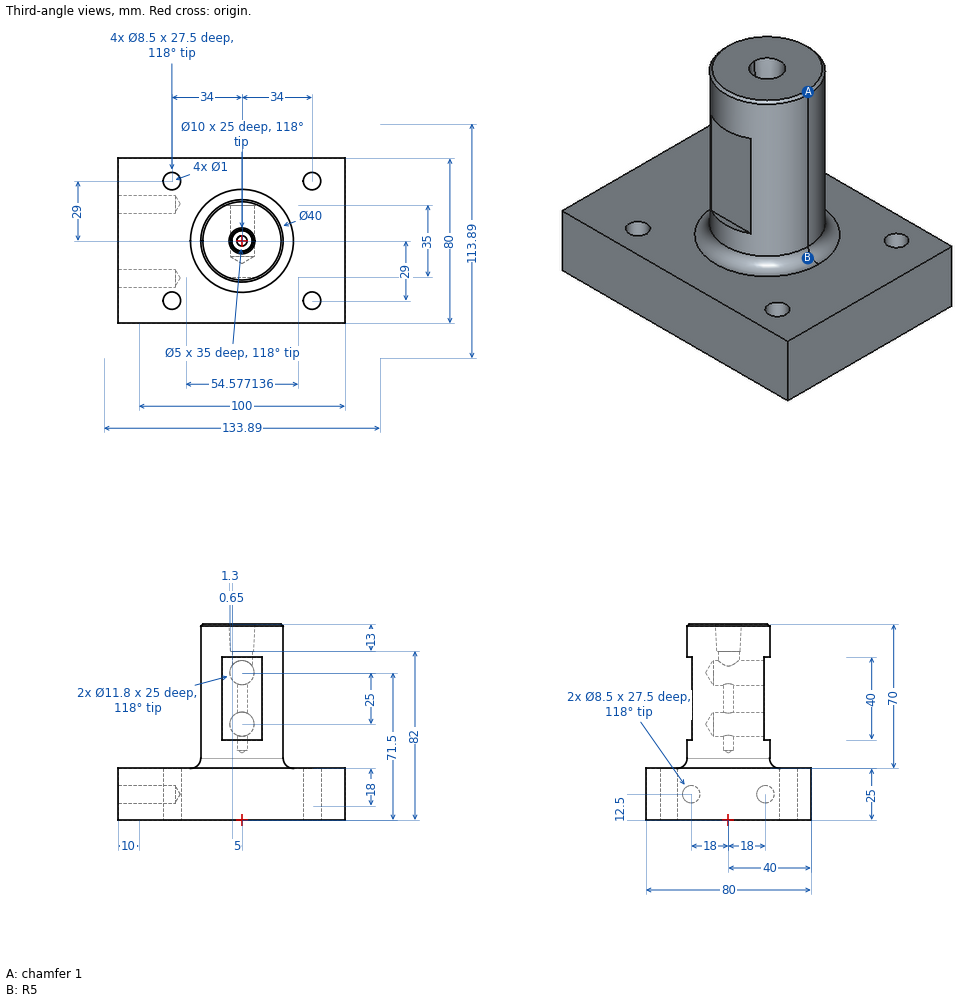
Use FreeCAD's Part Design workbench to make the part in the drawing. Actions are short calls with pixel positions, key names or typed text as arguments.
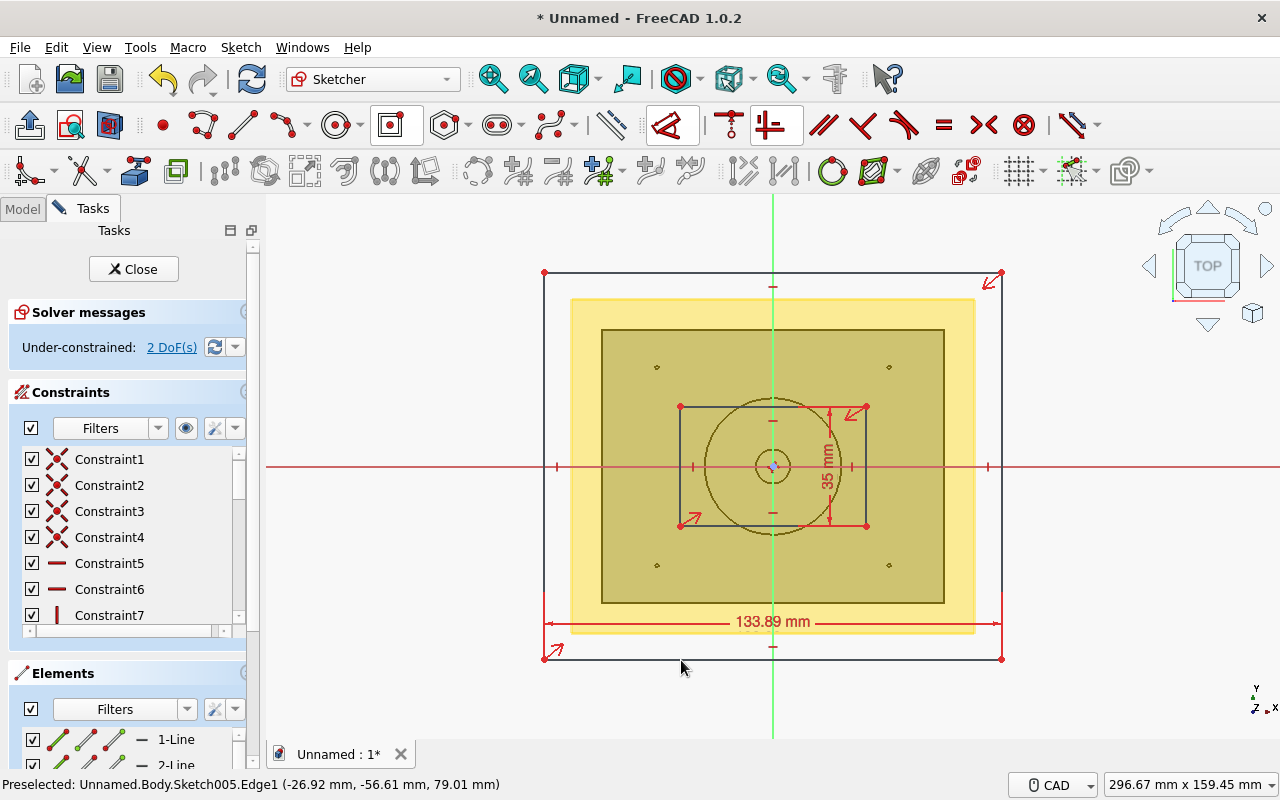
click(1002, 544)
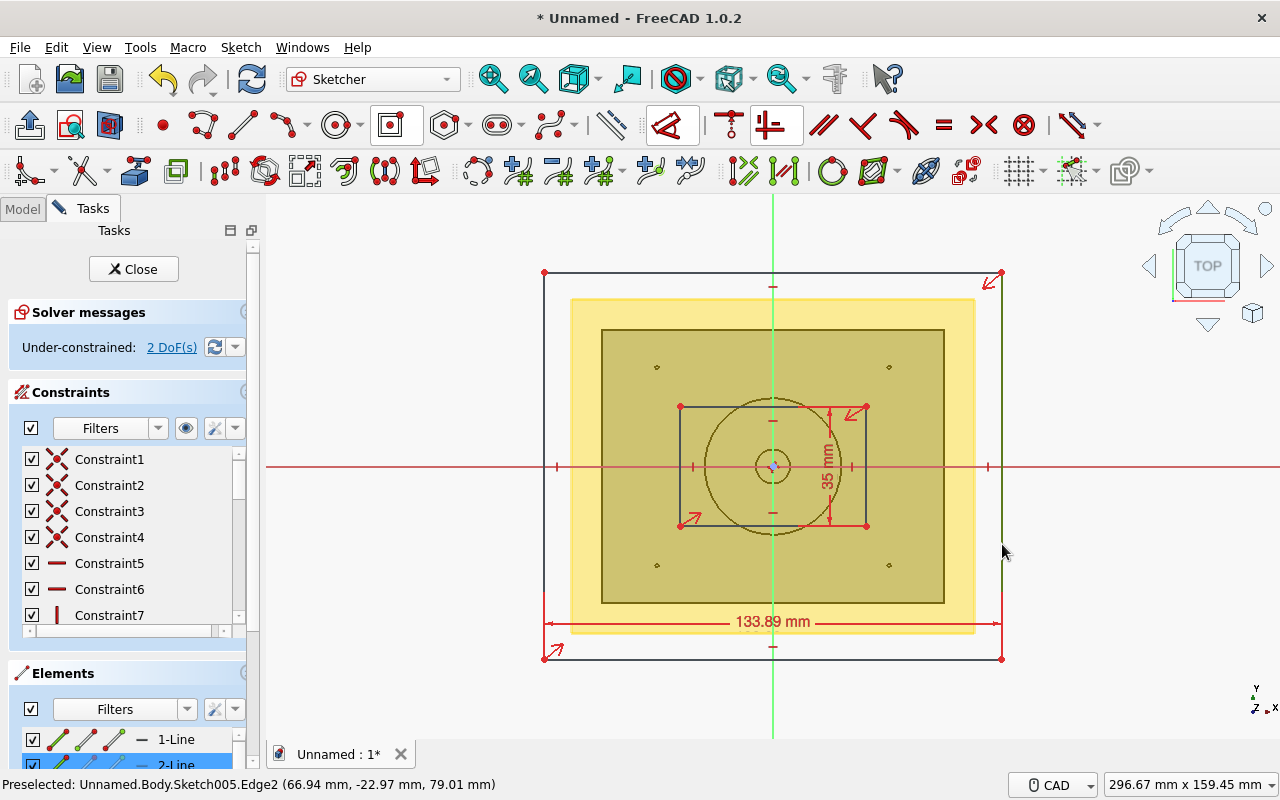
key(i)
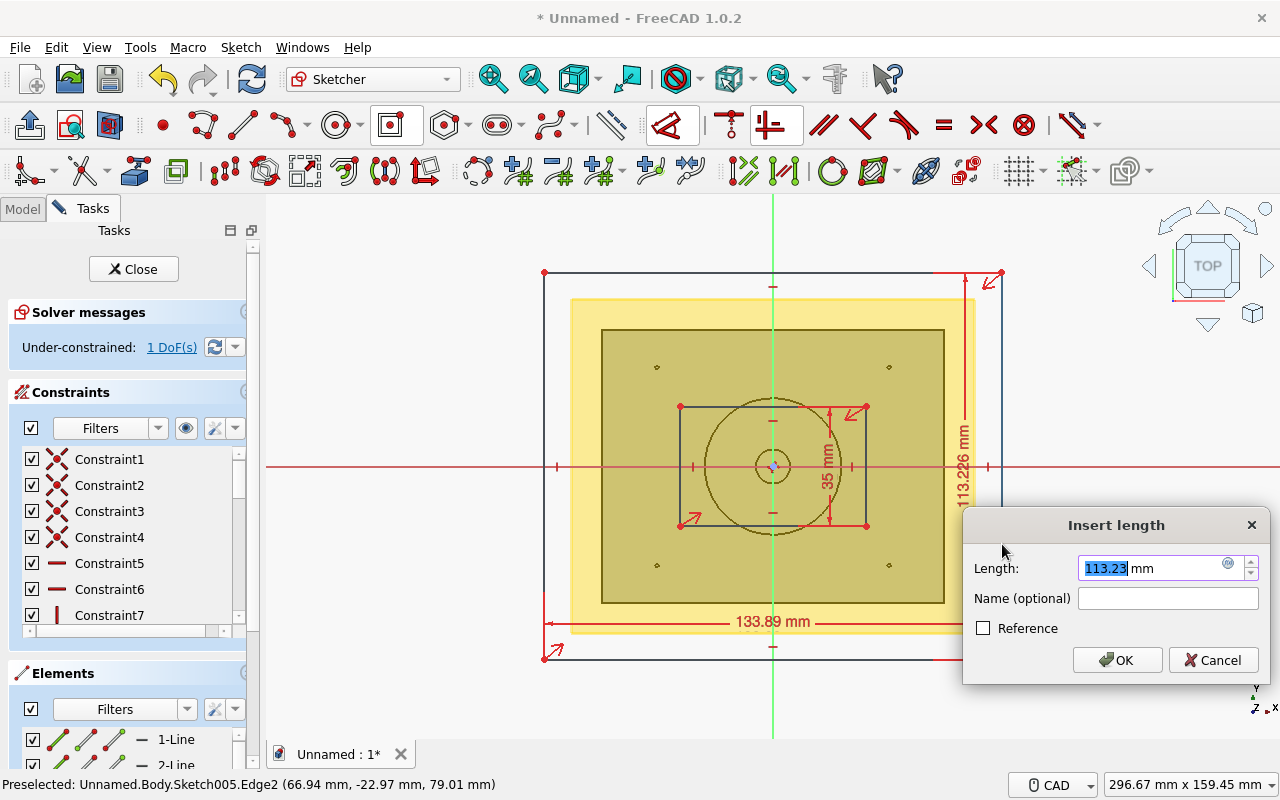
text(113.89)
key(Return)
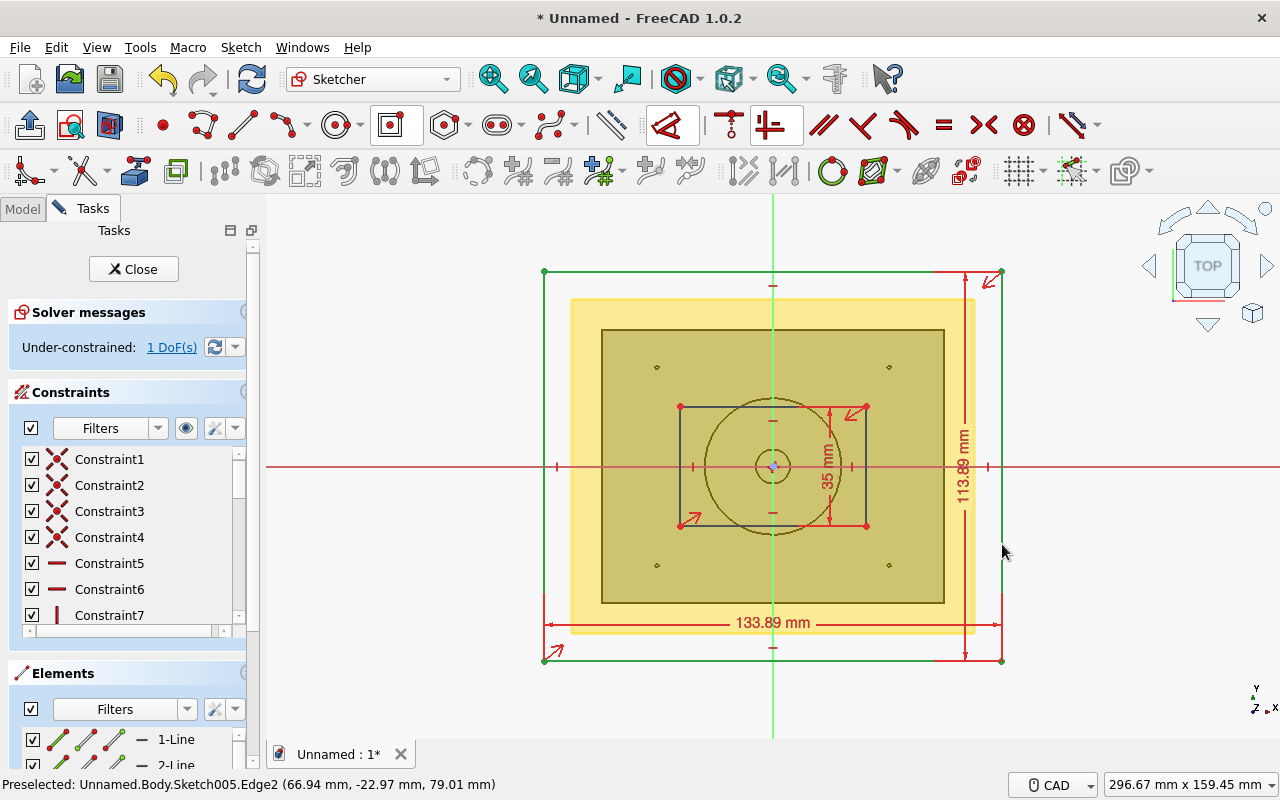
click(736, 526)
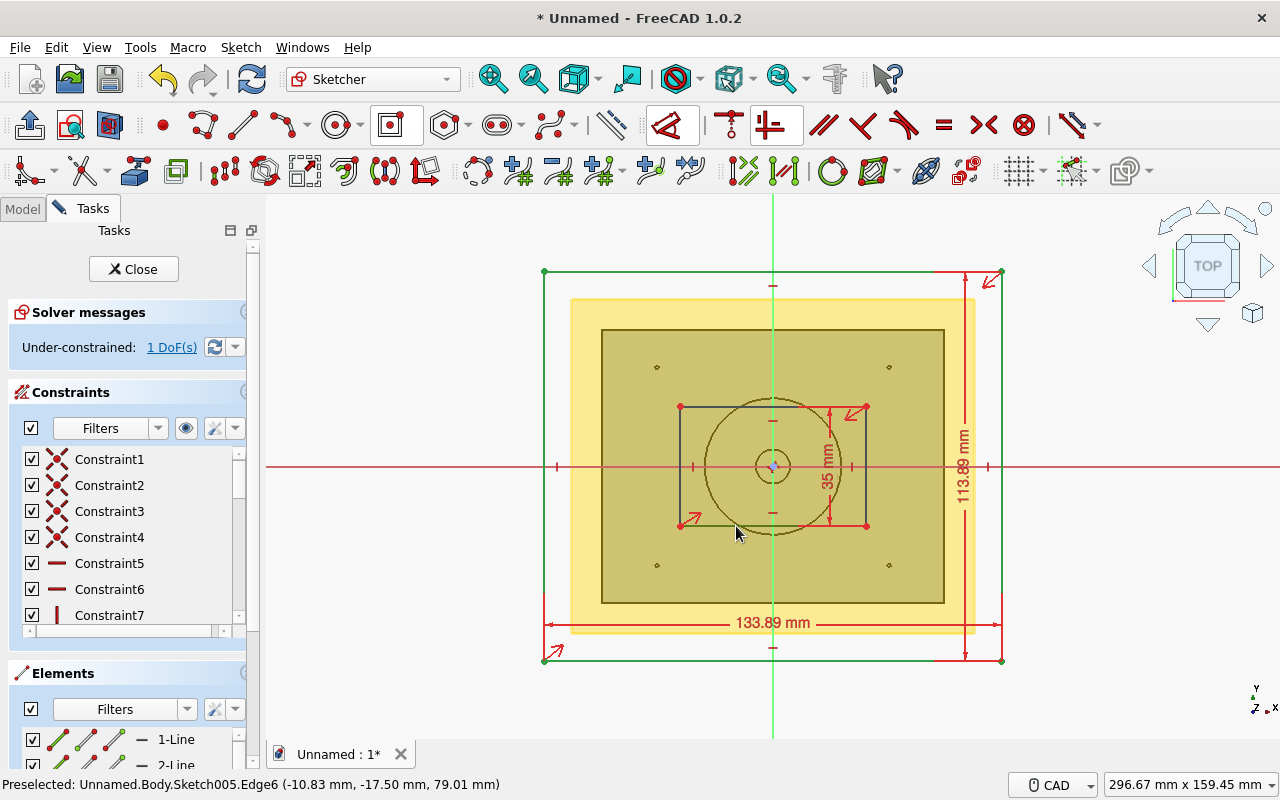
click(694, 126)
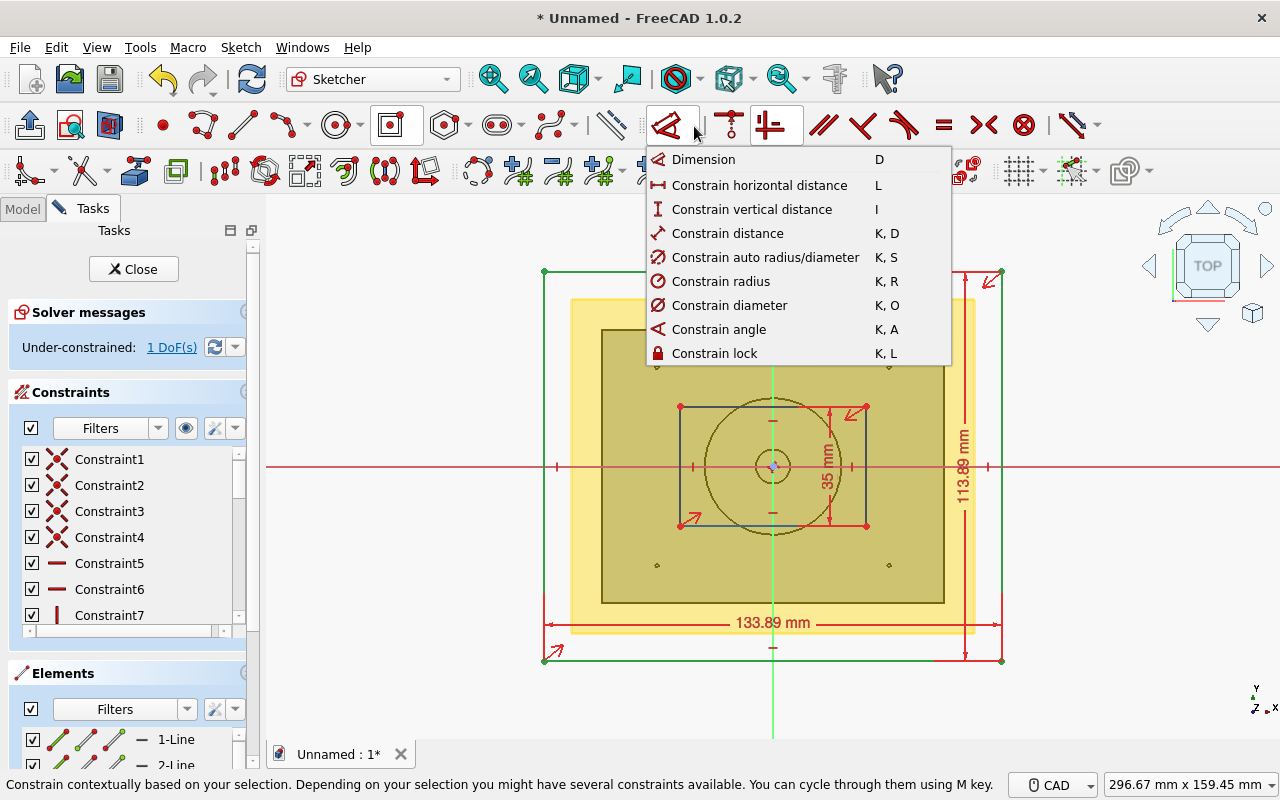
click(799, 185)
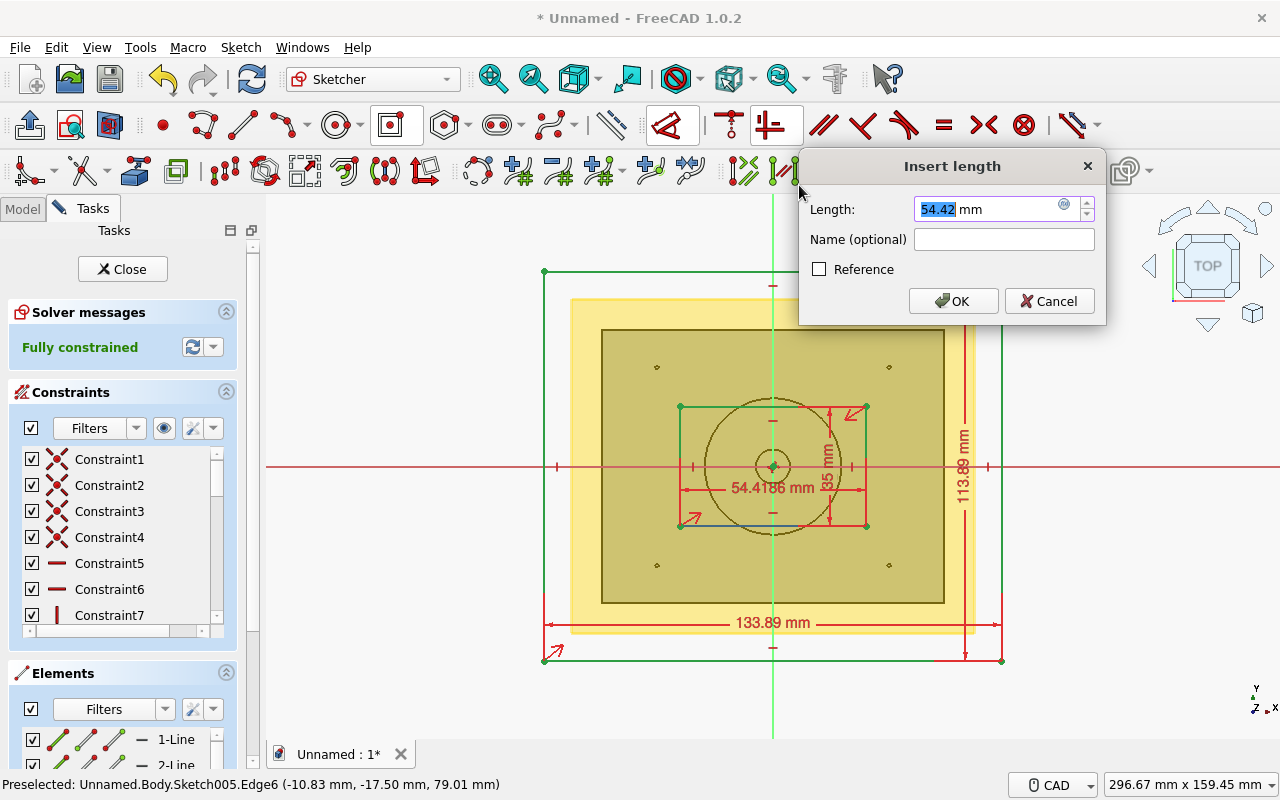
text(54.577136)
key(Return)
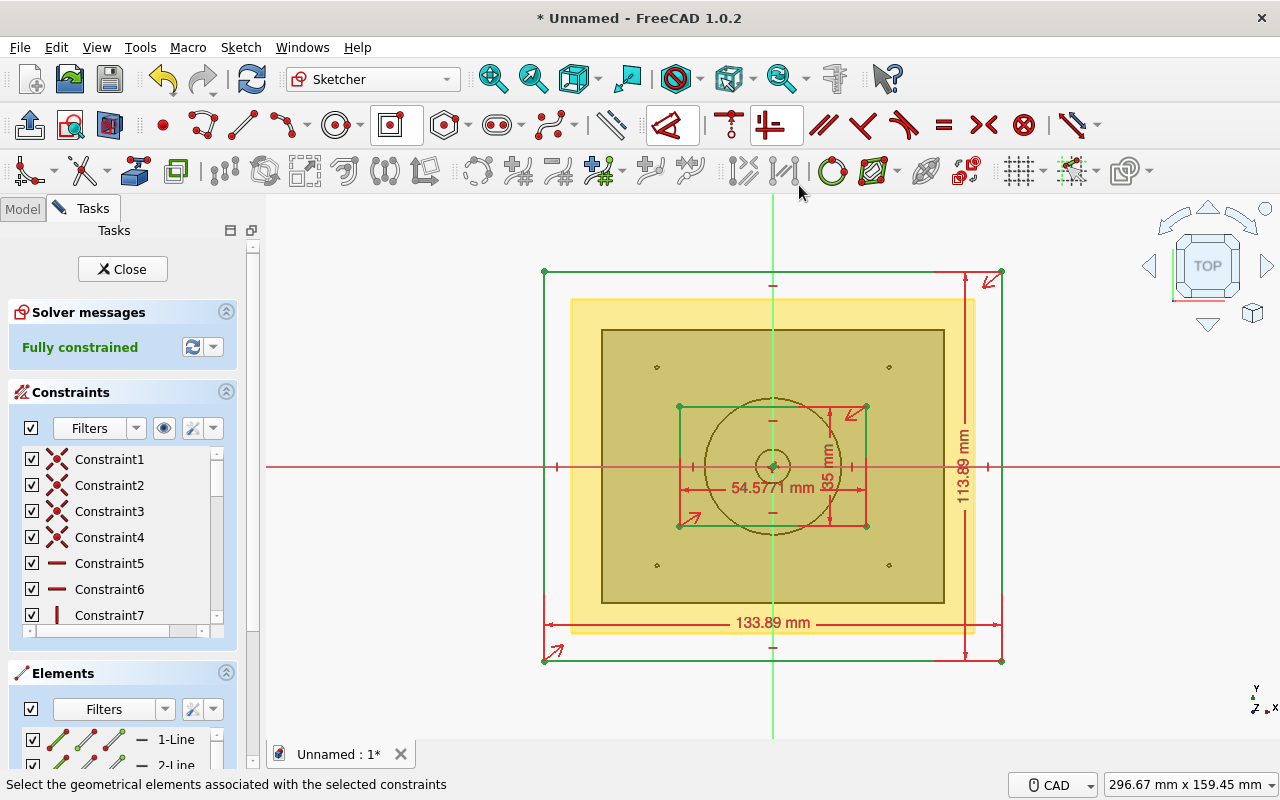
click(123, 269)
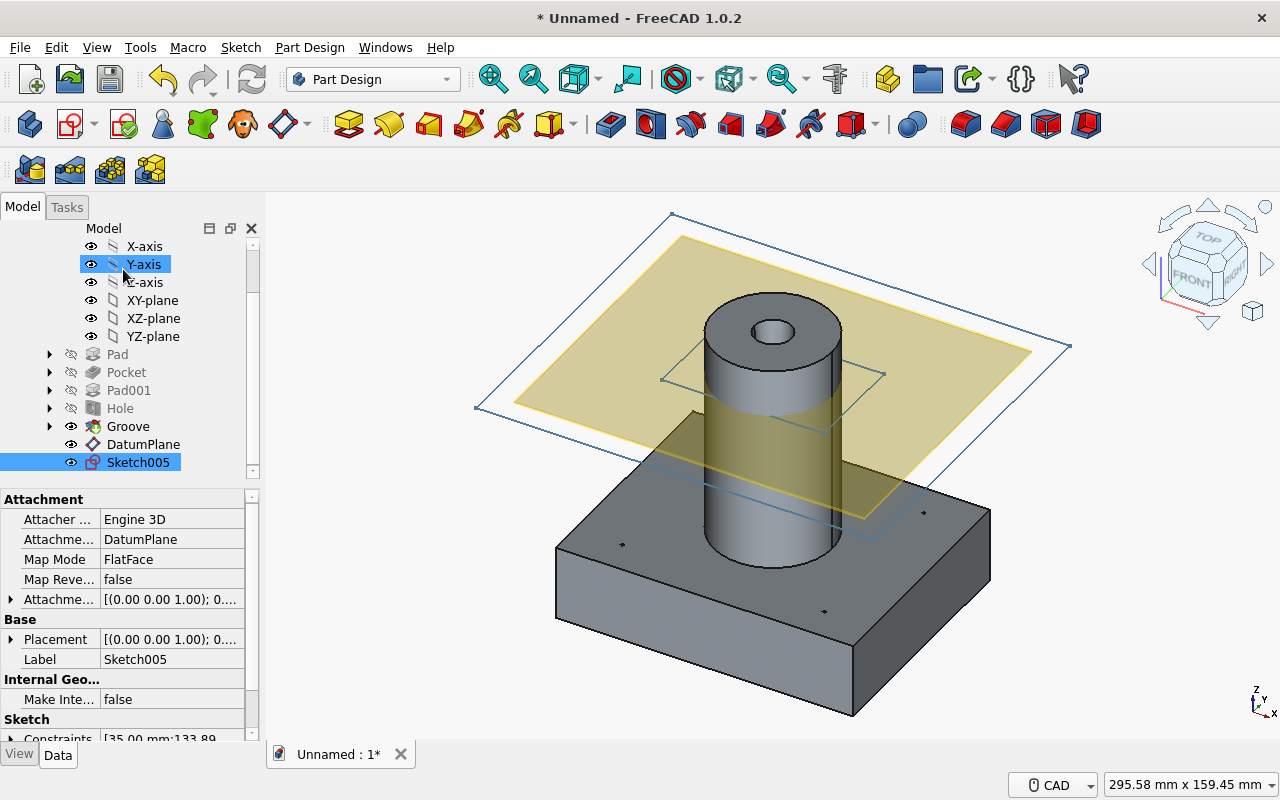
click(612, 124)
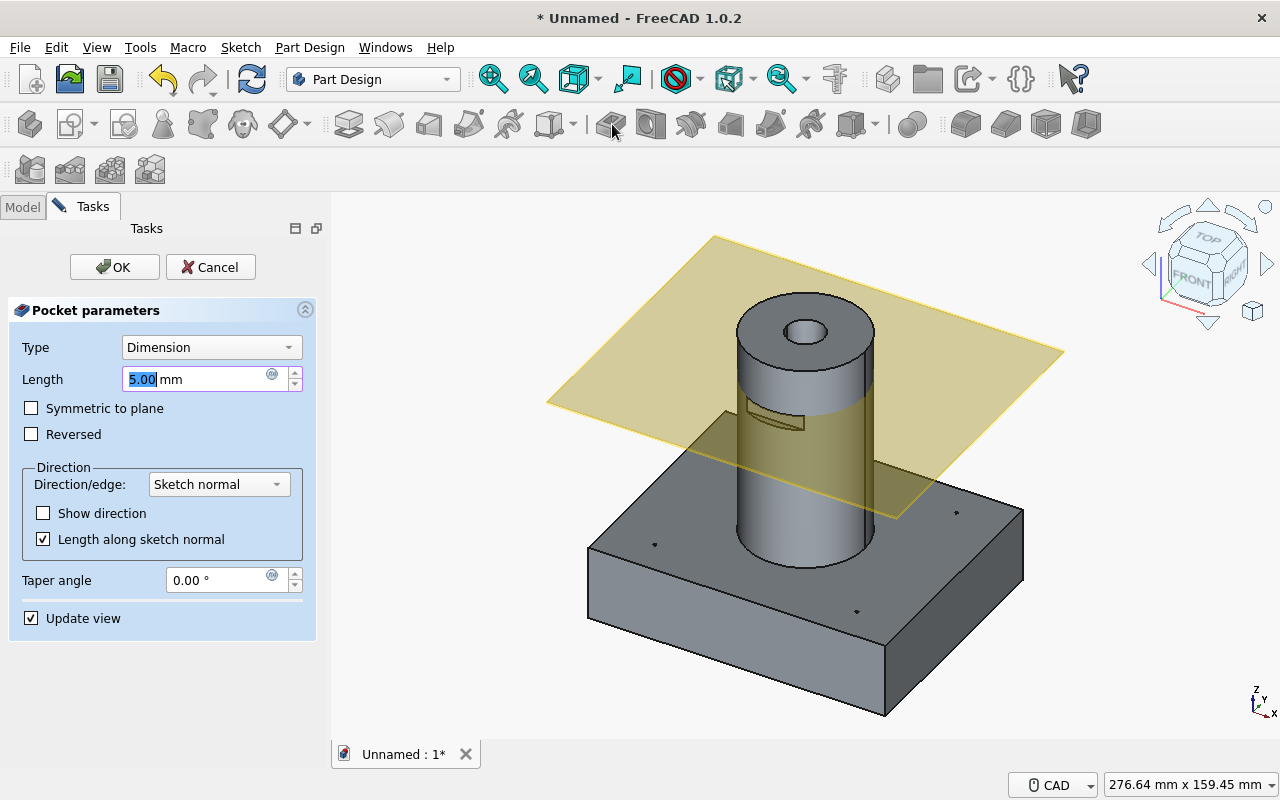
text(40)
key(Tab)